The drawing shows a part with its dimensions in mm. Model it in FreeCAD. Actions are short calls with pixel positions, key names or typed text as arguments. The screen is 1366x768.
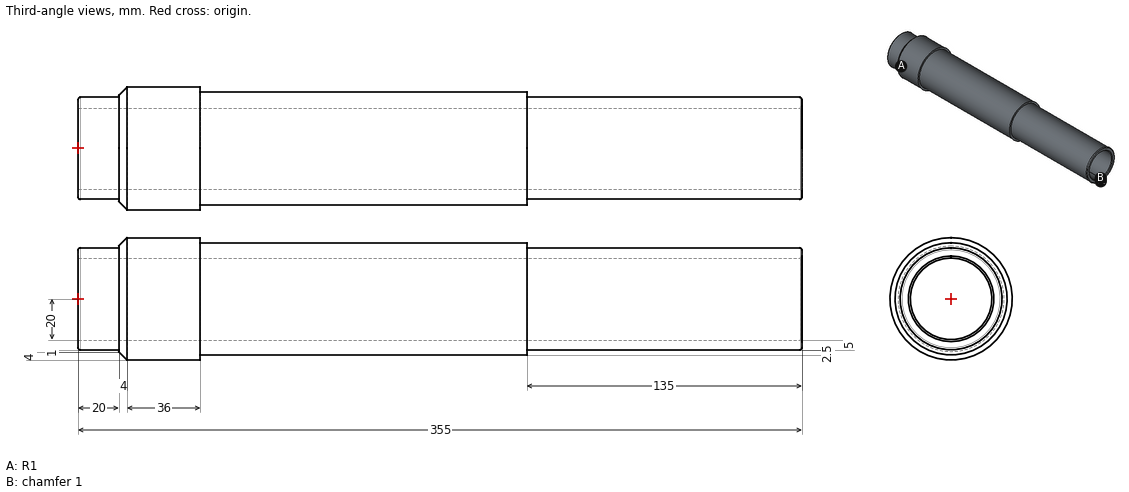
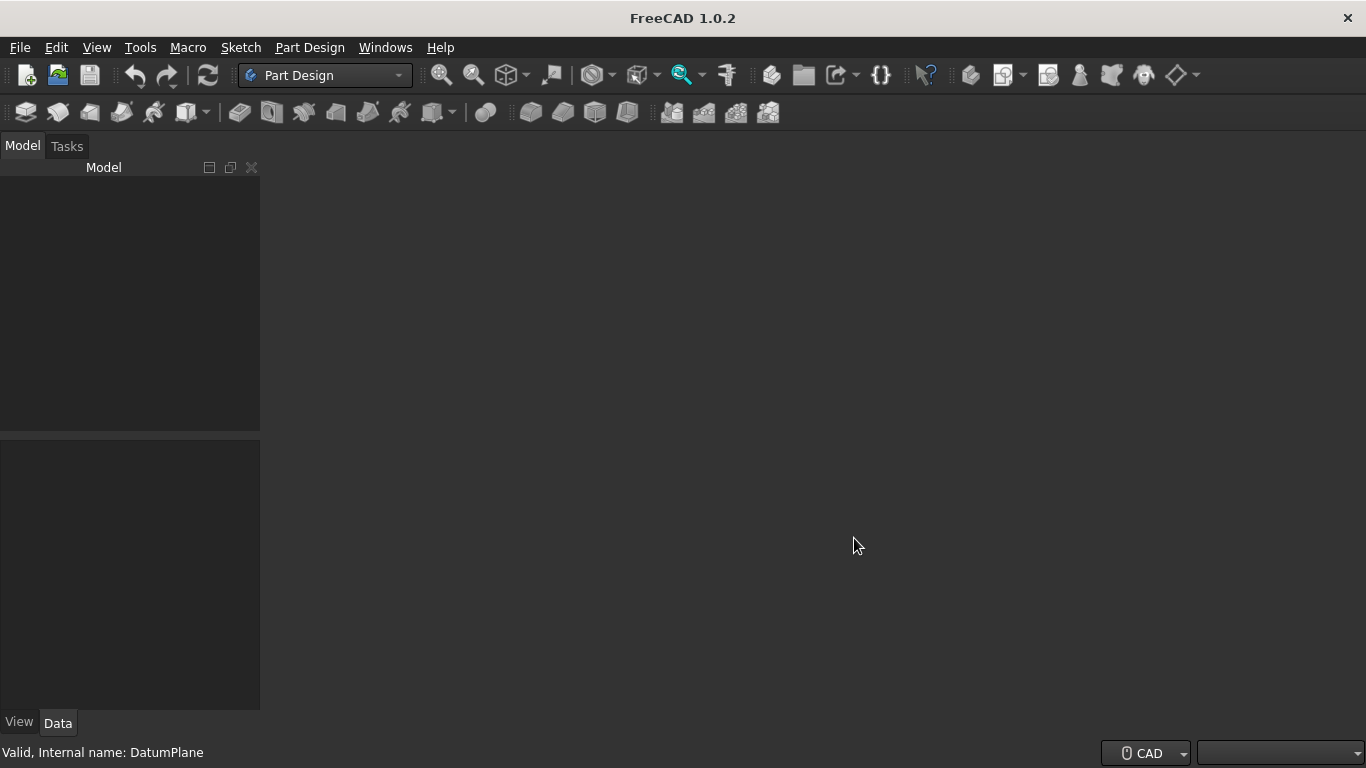
key(ctrl+n)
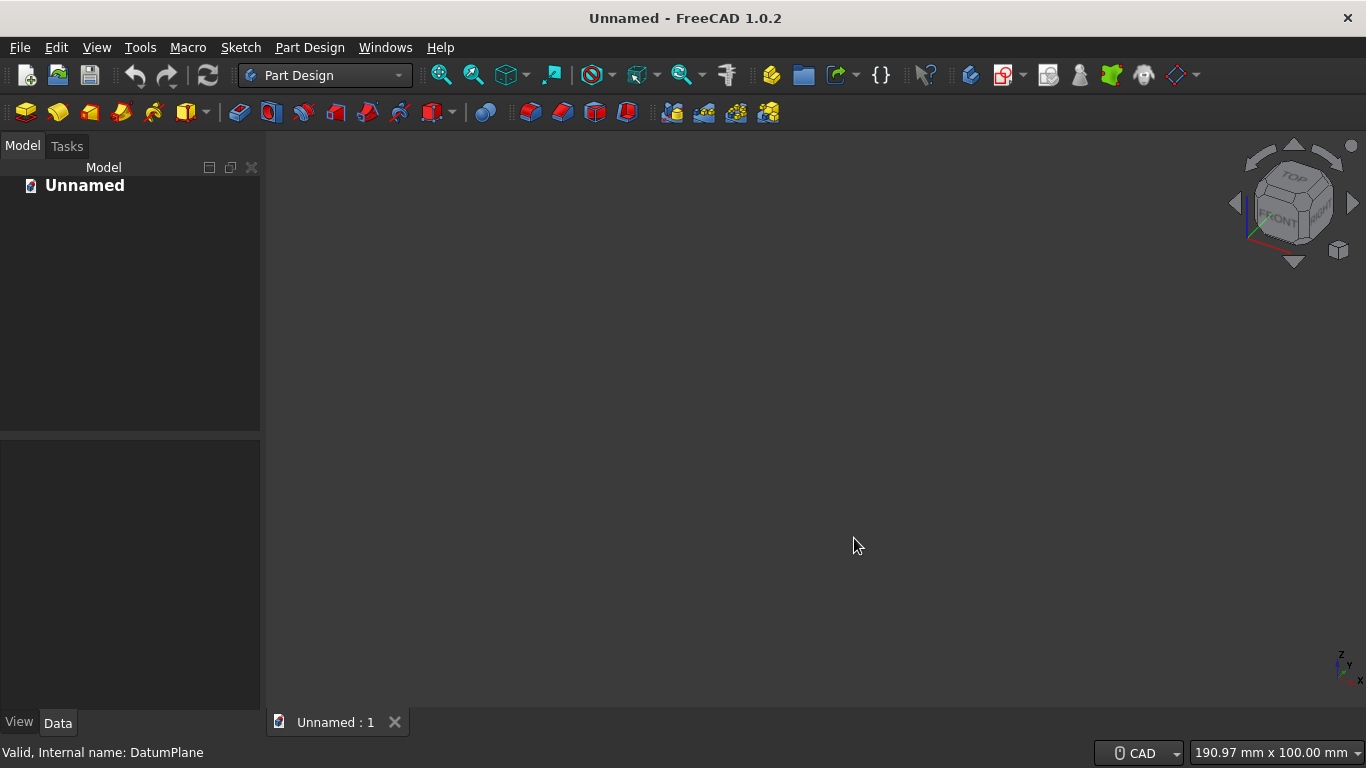
click(1004, 76)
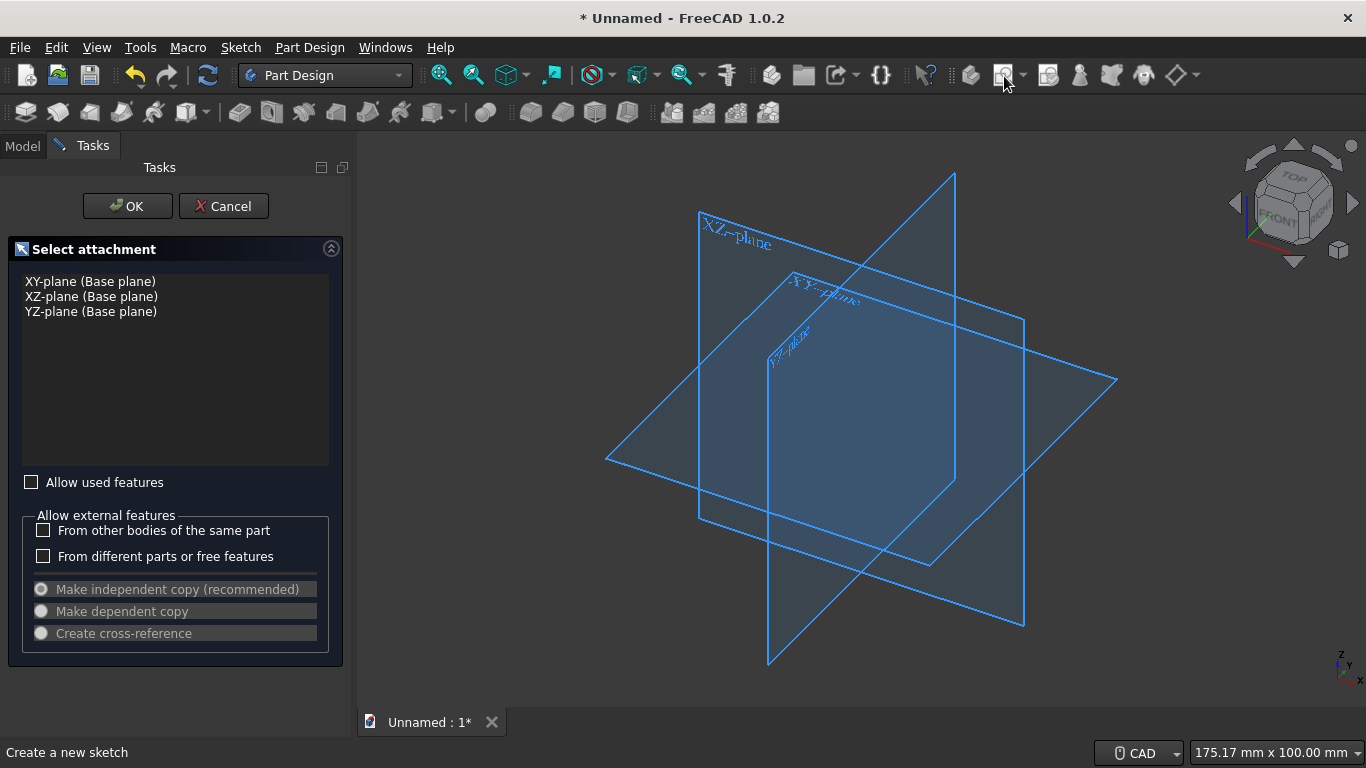
click(82, 296)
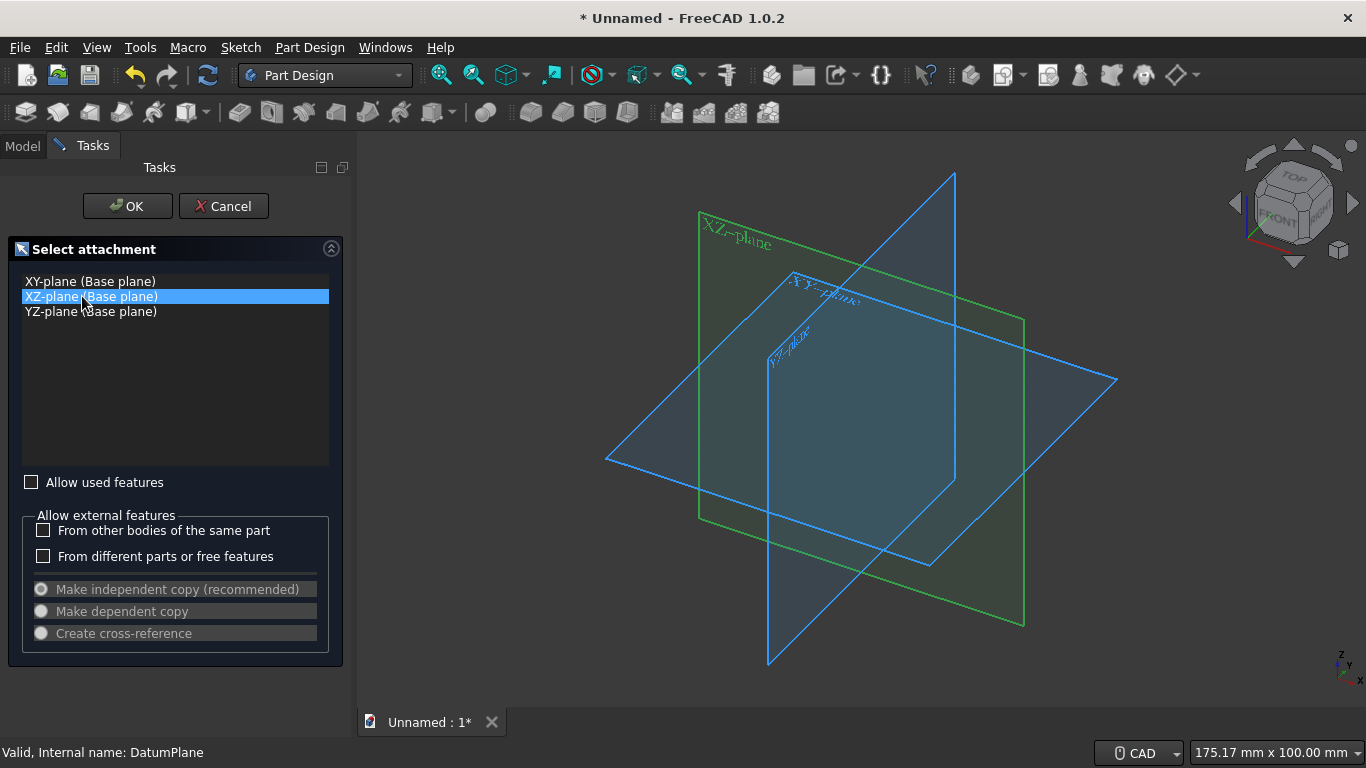
click(128, 206)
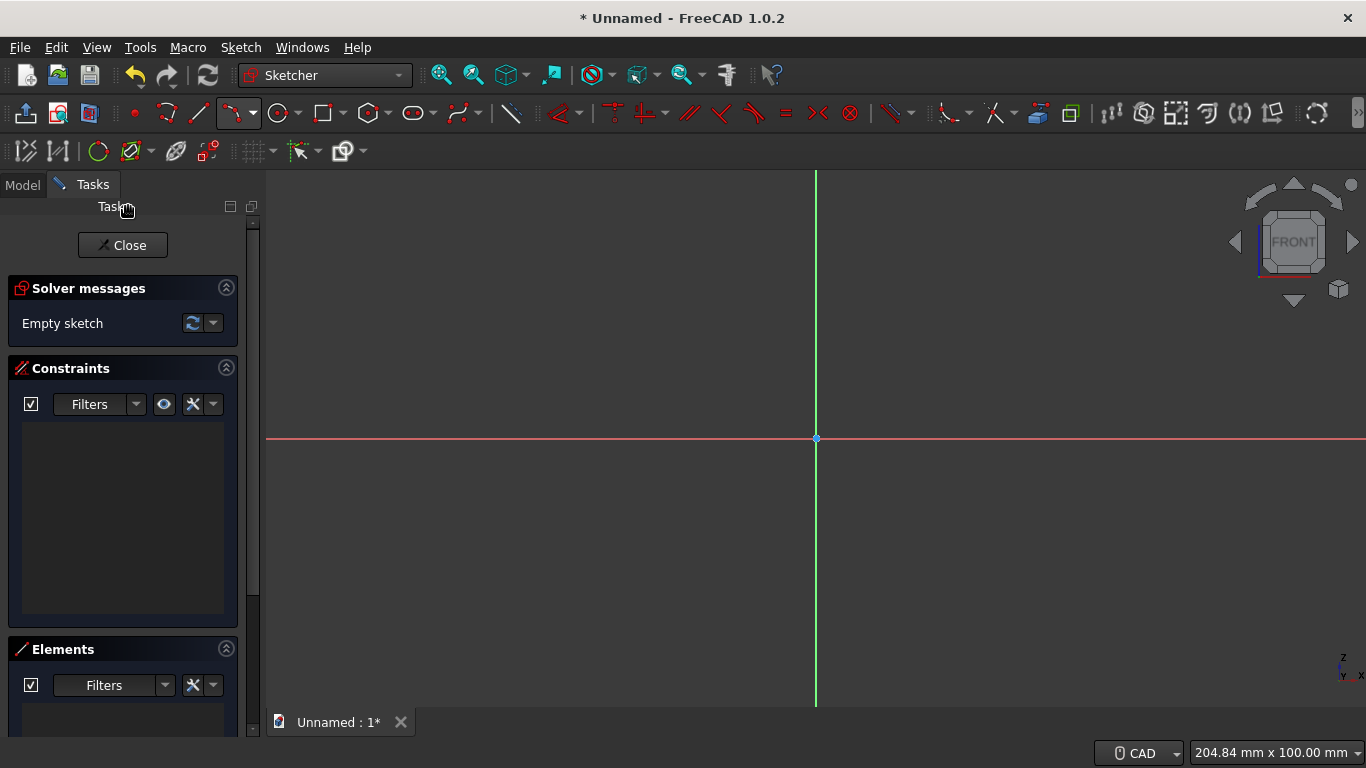
scroll(307, 404, down, 6)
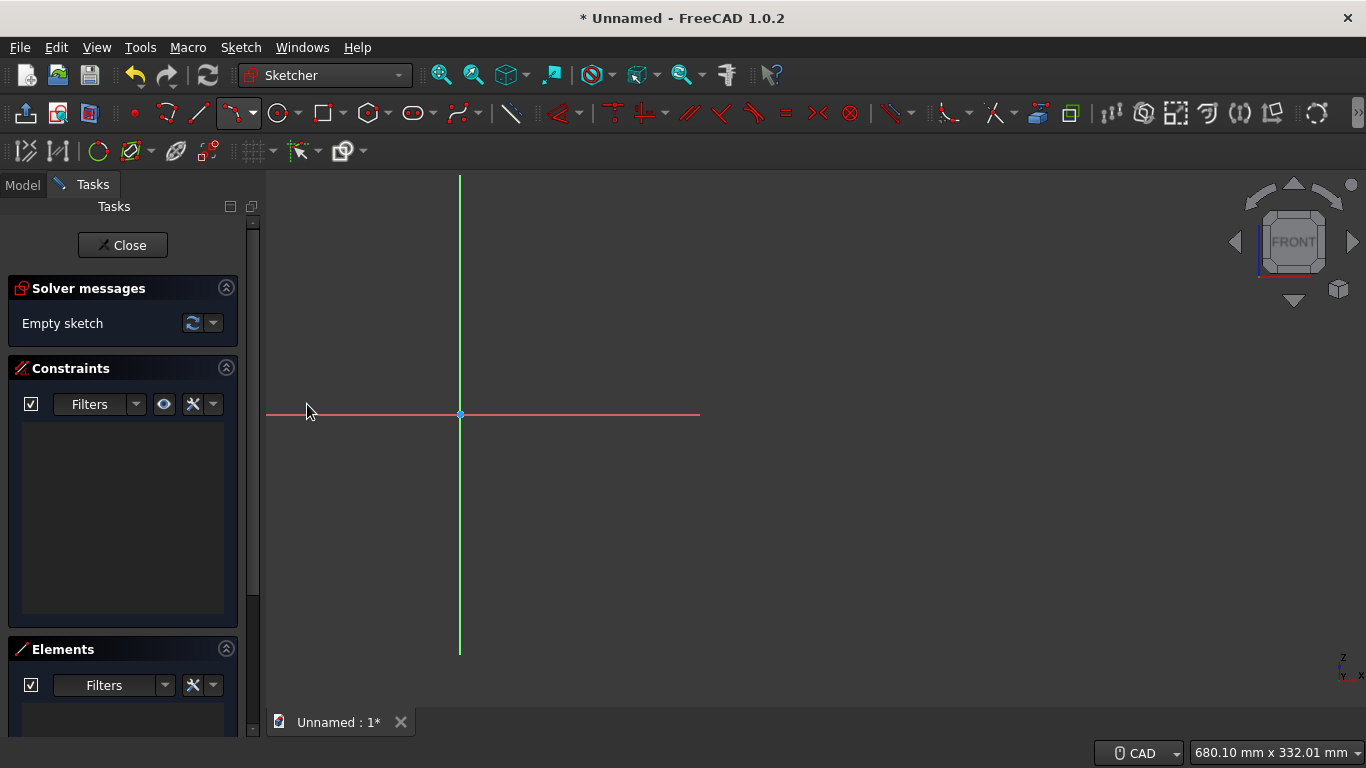
key(g)
key(m)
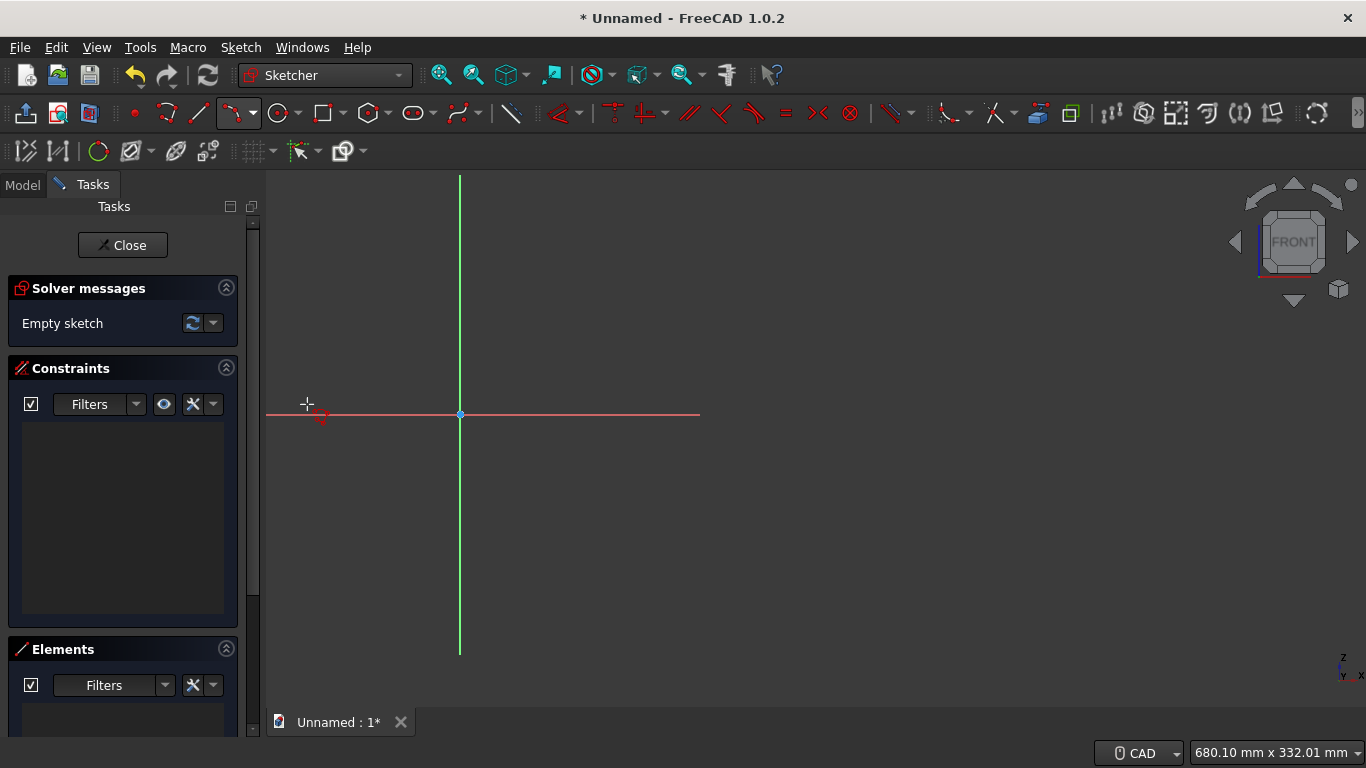
click(460, 447)
click(1035, 447)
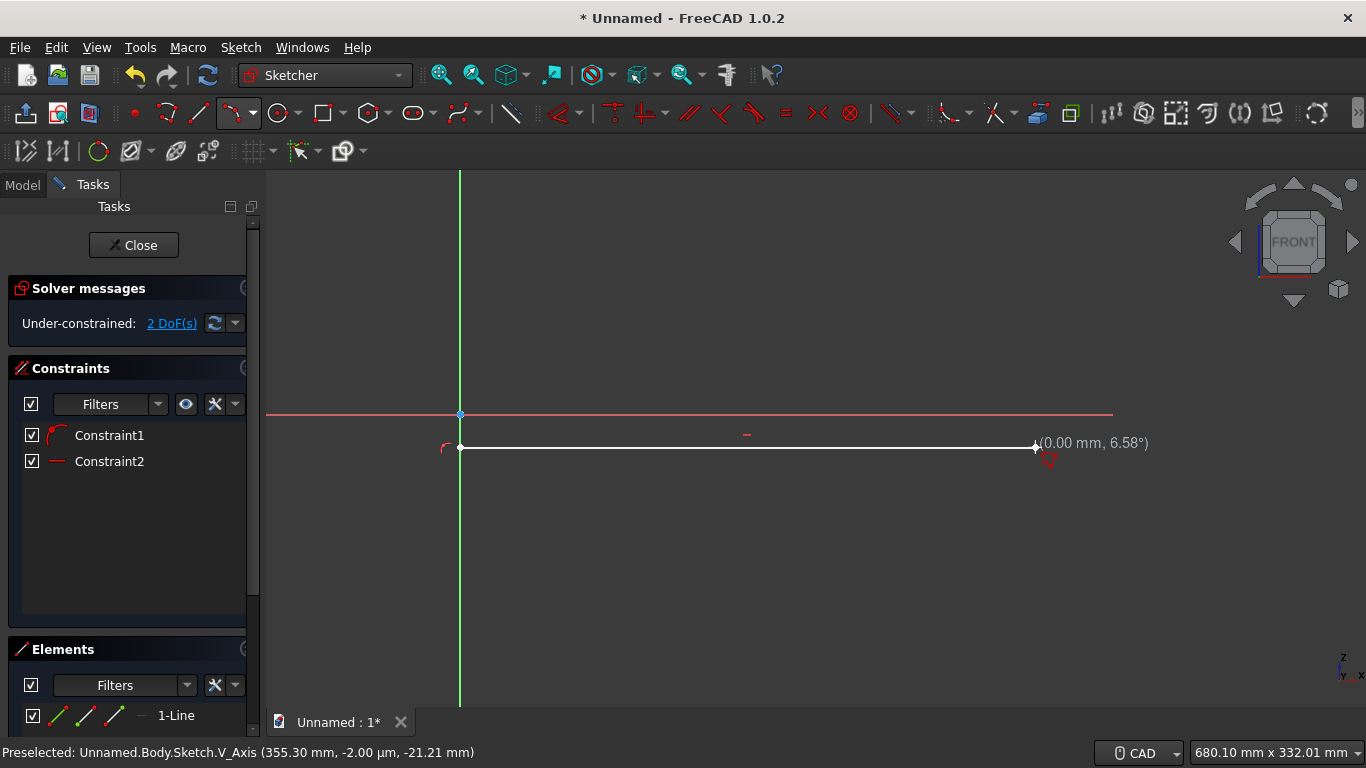
scroll(1035, 455, up, 4)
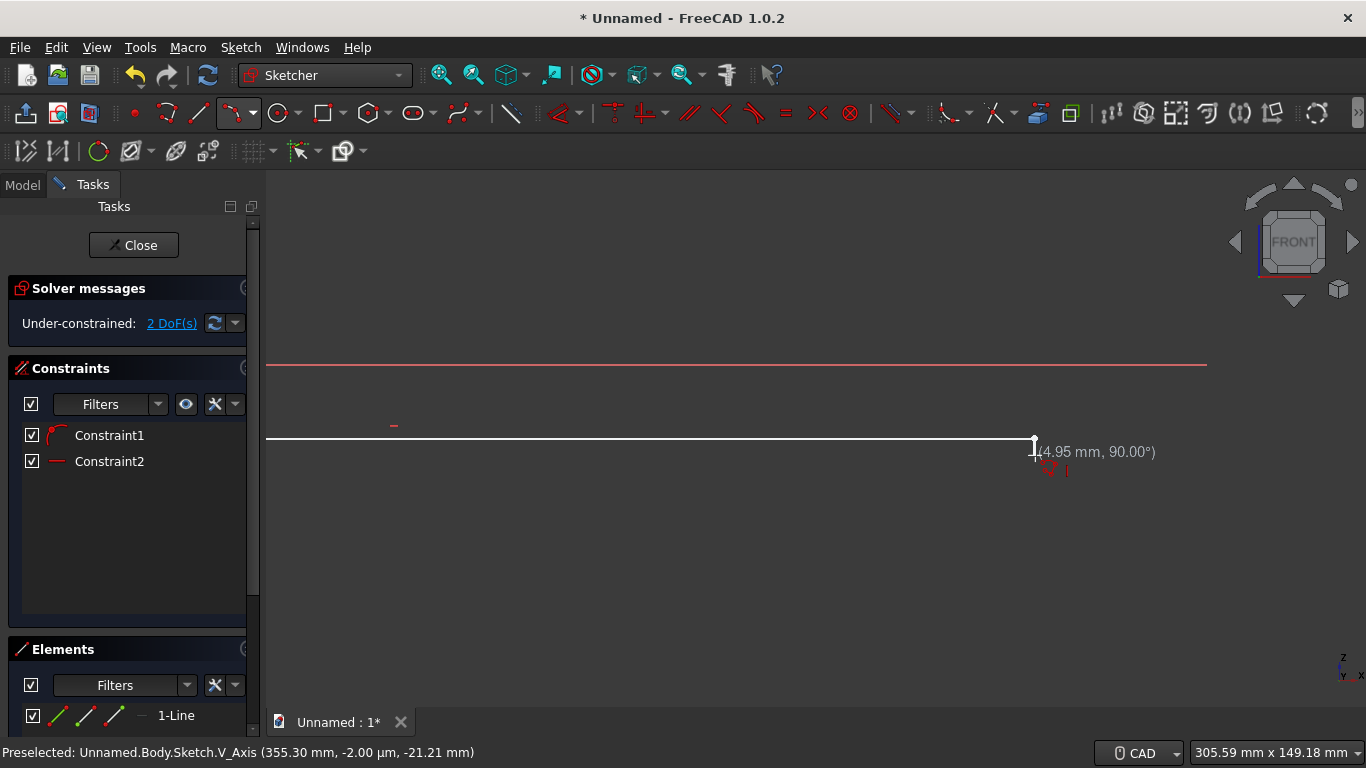
click(1034, 455)
click(547, 455)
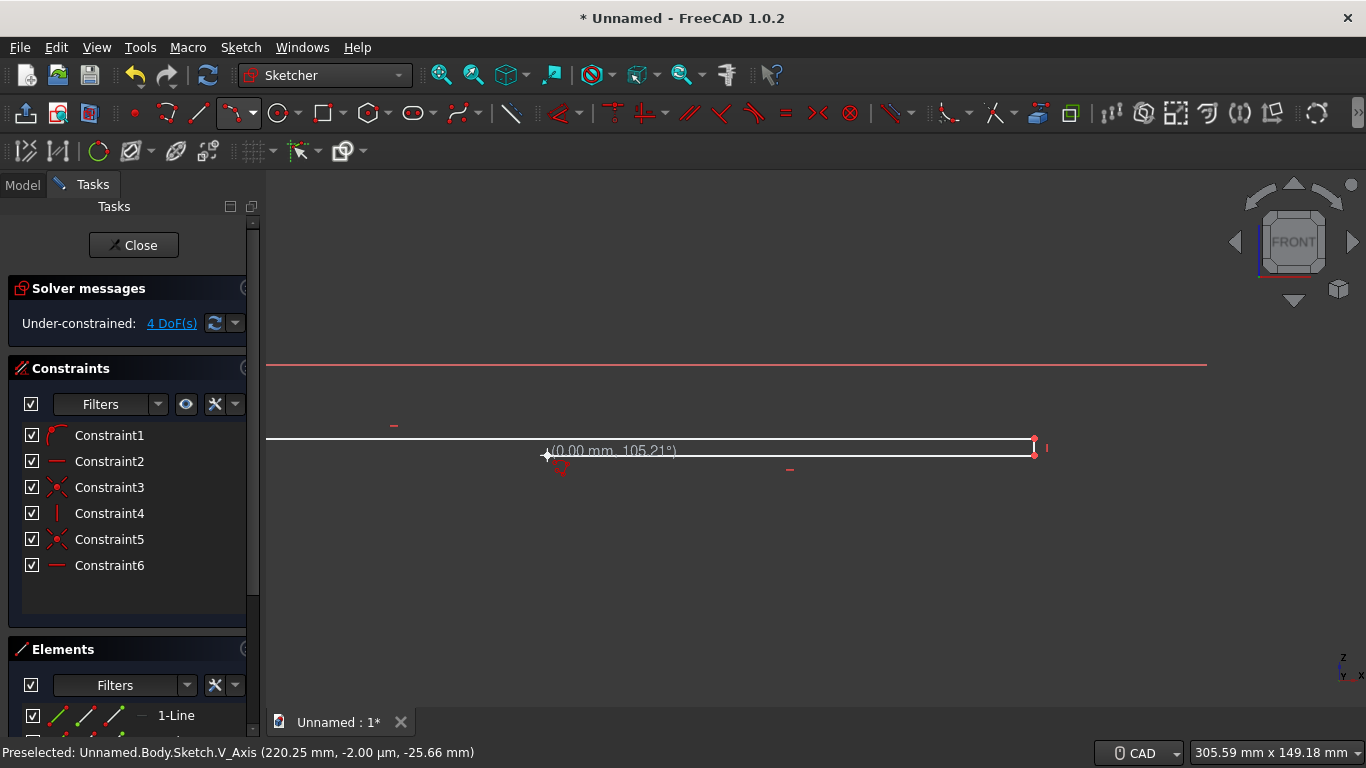
scroll(547, 464, up, 3)